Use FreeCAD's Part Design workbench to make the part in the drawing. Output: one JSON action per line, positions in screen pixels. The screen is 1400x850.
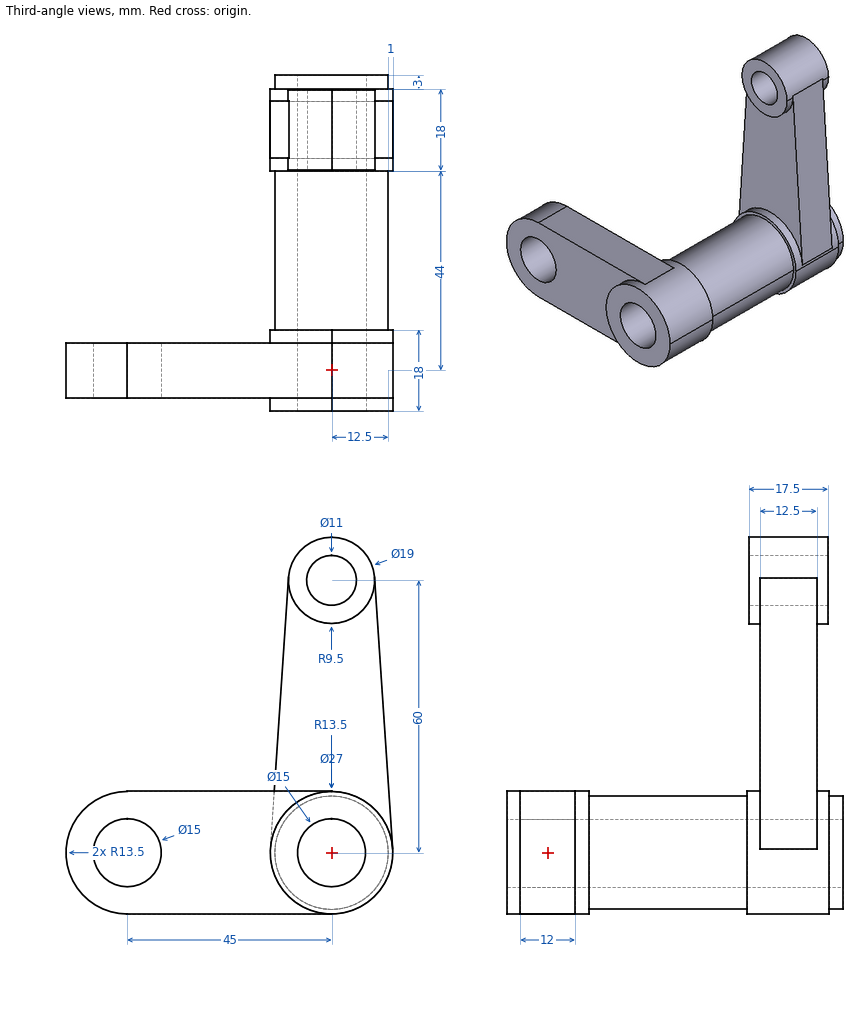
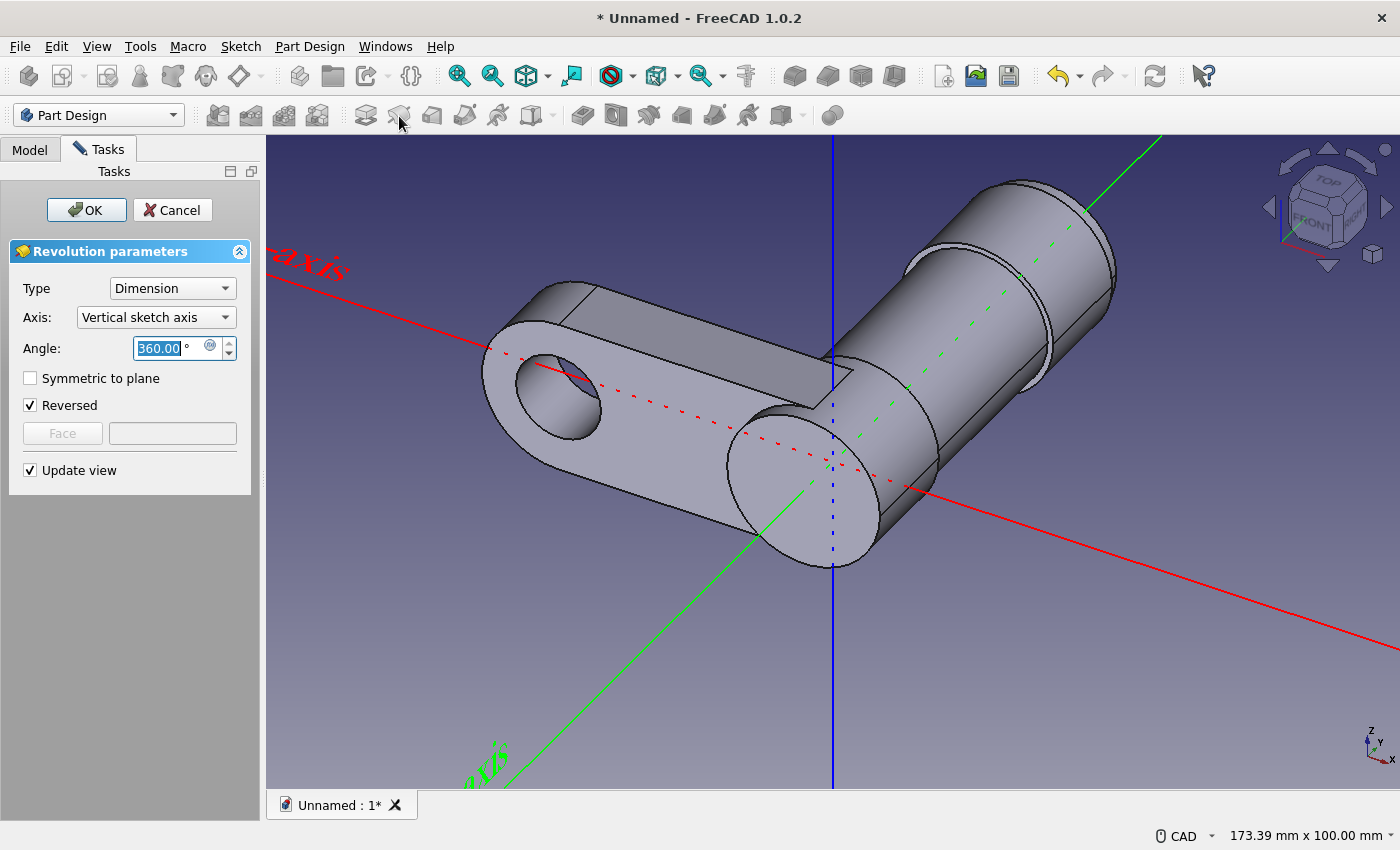
{"action": "left_click", "coordinate": [87, 210]}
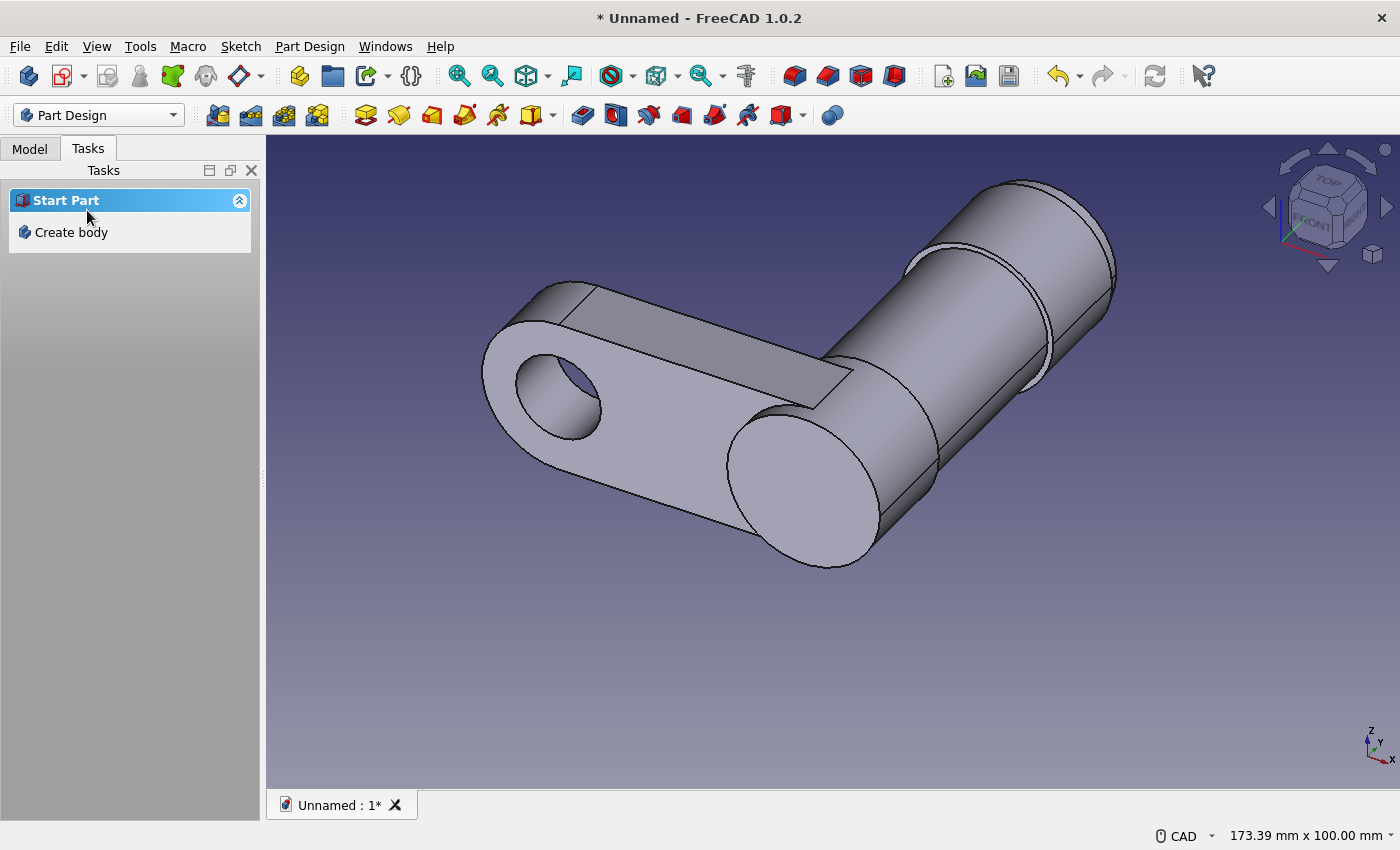
{"action": "key", "text": "v f"}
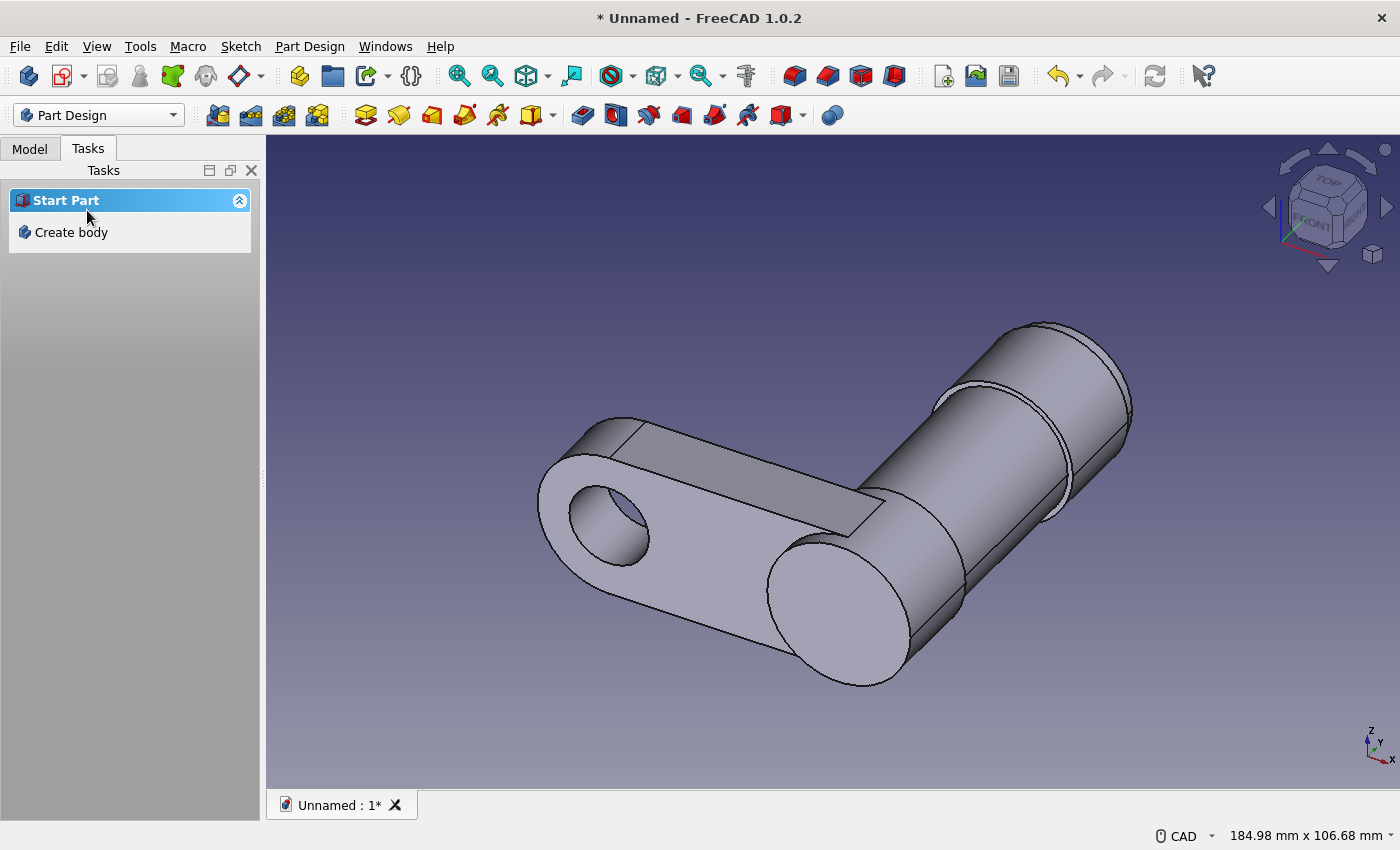
{"action": "key", "text": "4"}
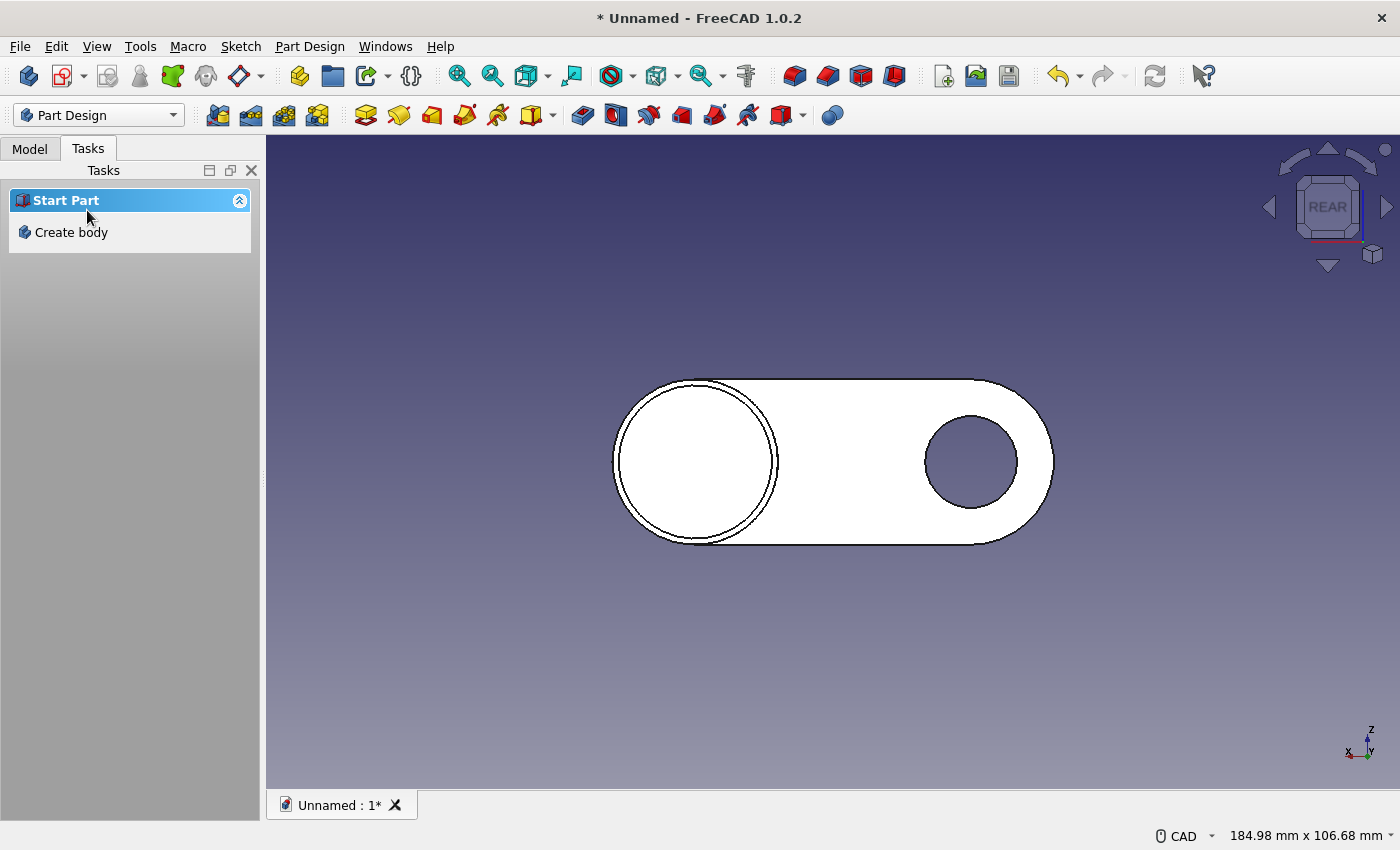
{"action": "key", "text": "v f"}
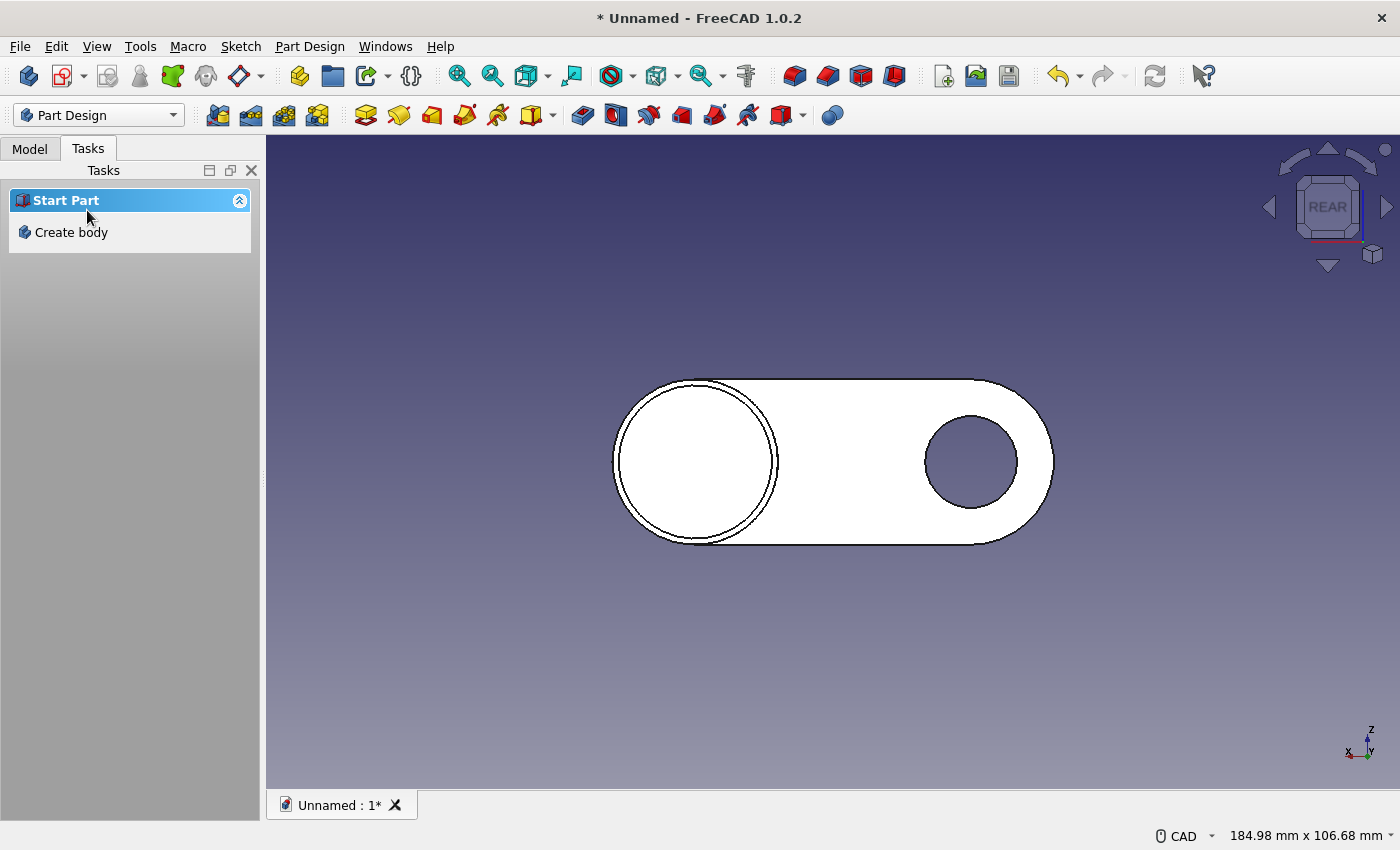
{"action": "left_click", "coordinate": [695, 461]}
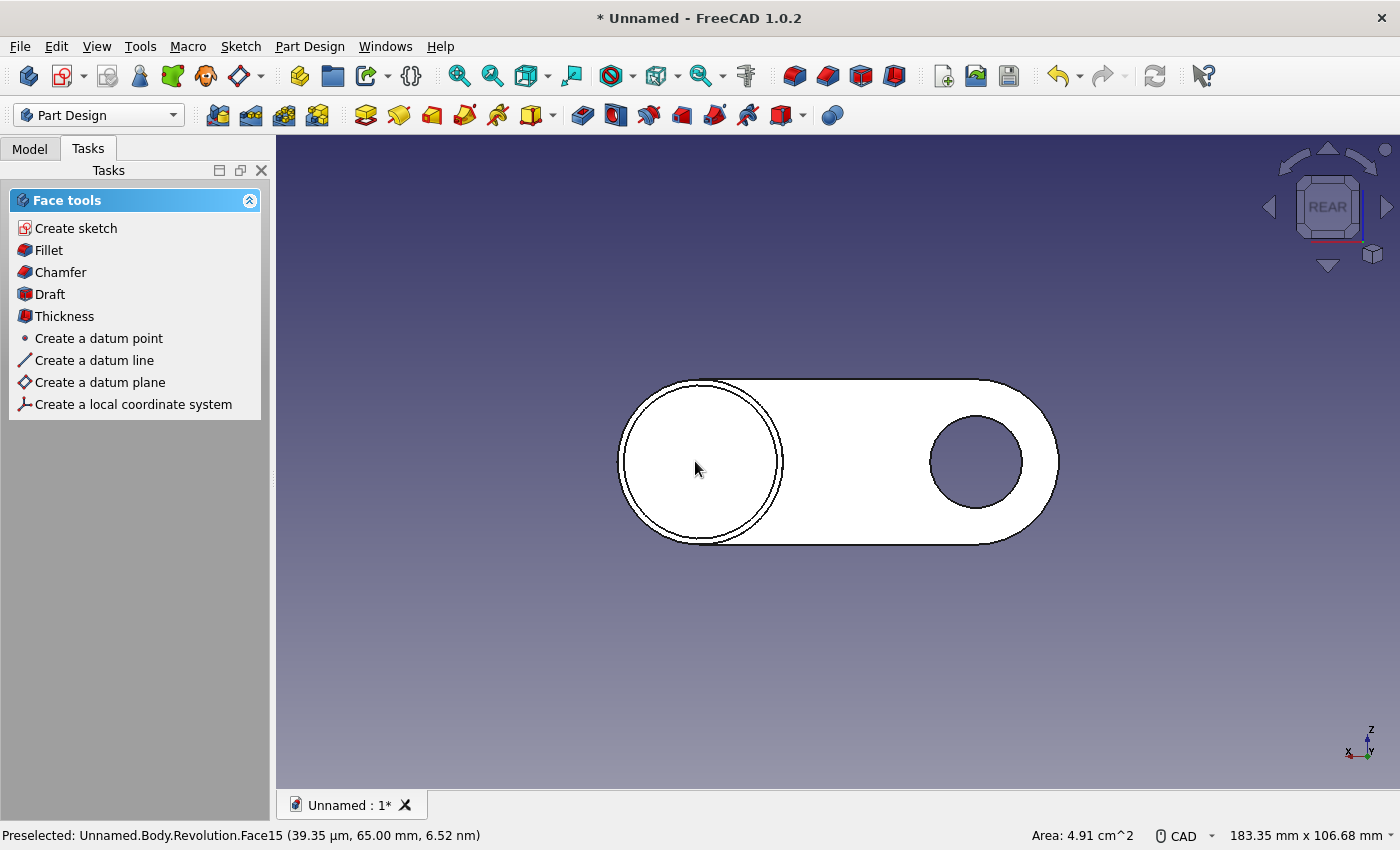
{"action": "left_click", "coordinate": [62, 76]}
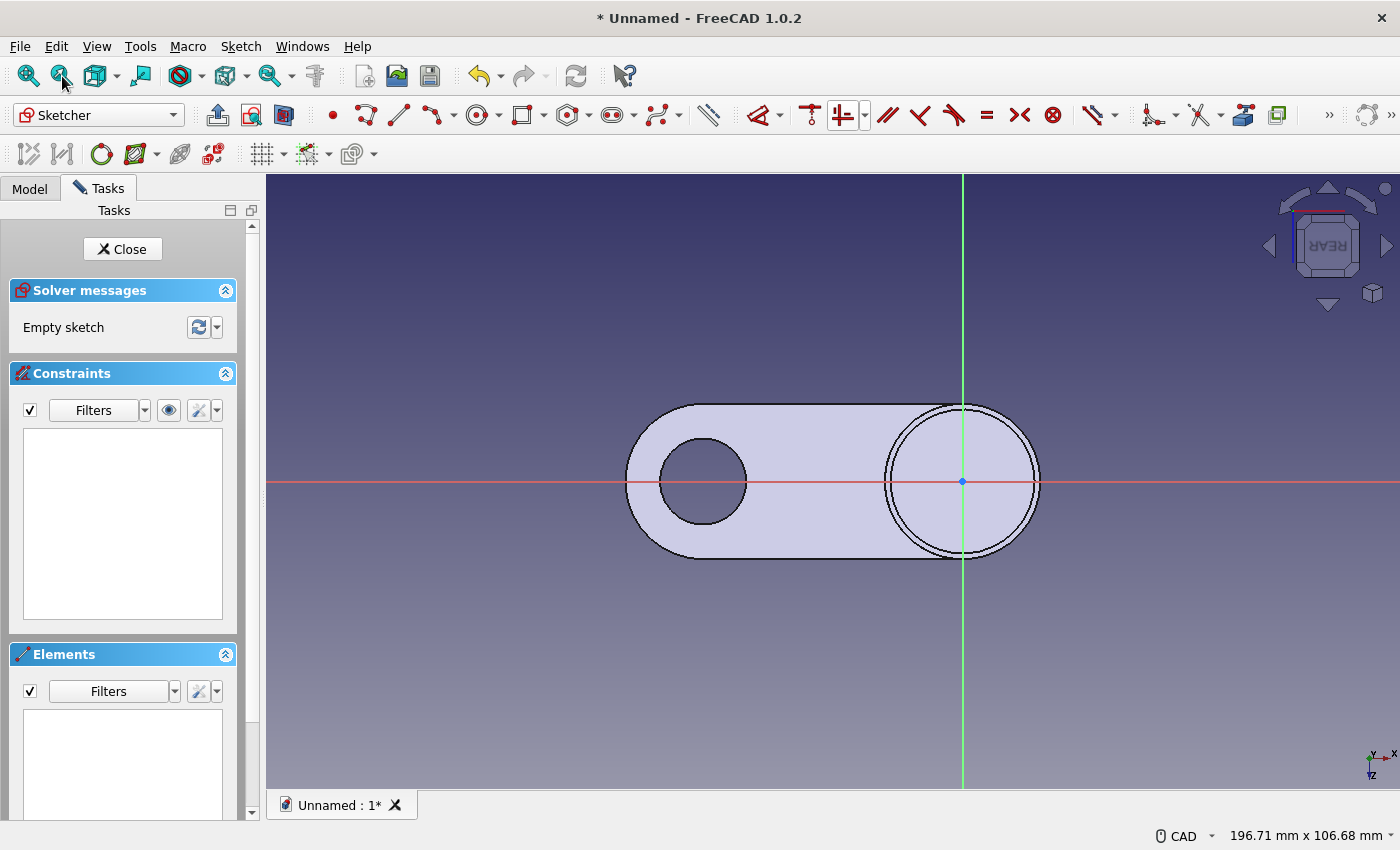
{"action": "scroll", "coordinate": [1013, 481], "scroll_direction": "up", "scroll_amount": 8}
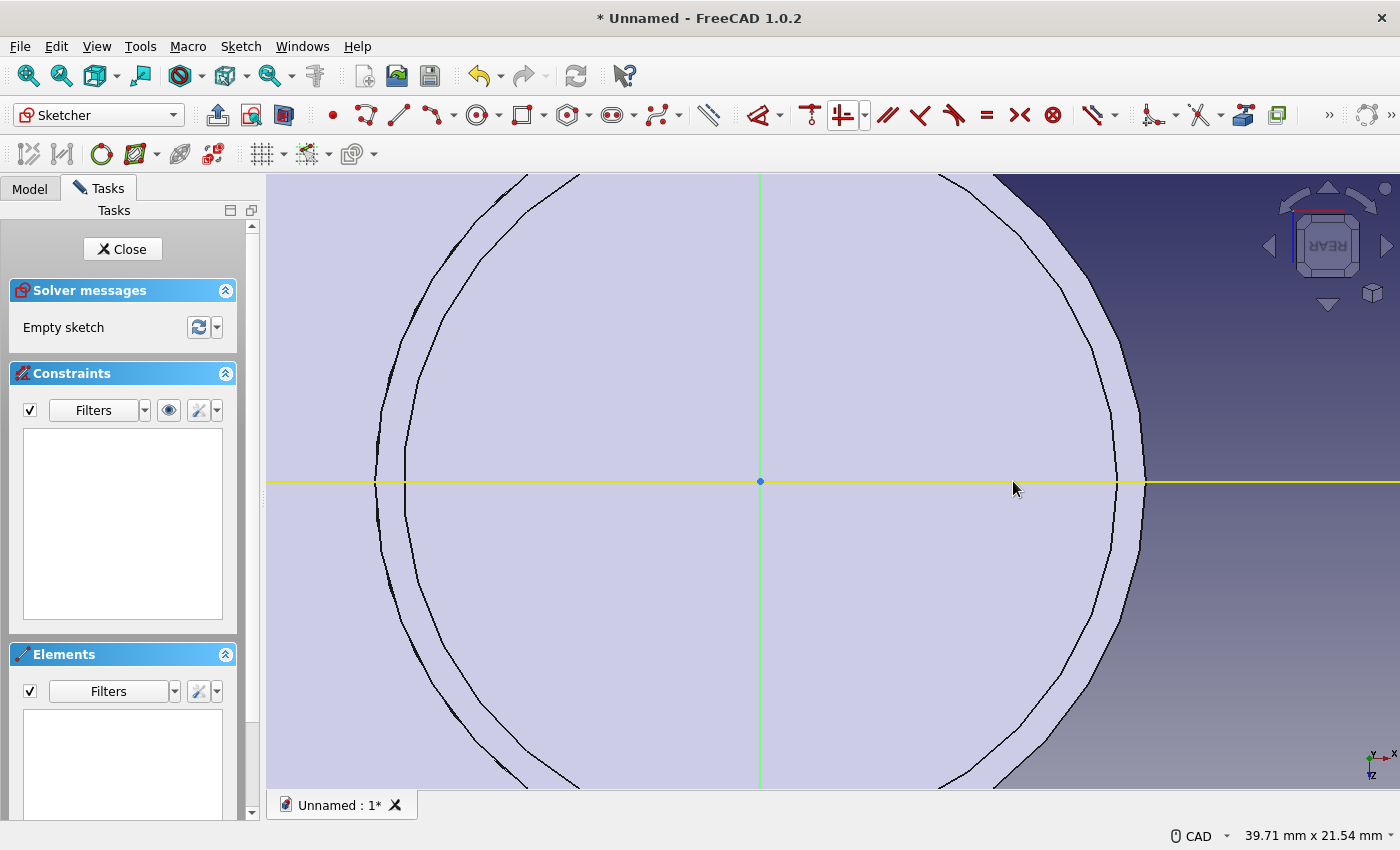
{"action": "left_click", "coordinate": [476, 116]}